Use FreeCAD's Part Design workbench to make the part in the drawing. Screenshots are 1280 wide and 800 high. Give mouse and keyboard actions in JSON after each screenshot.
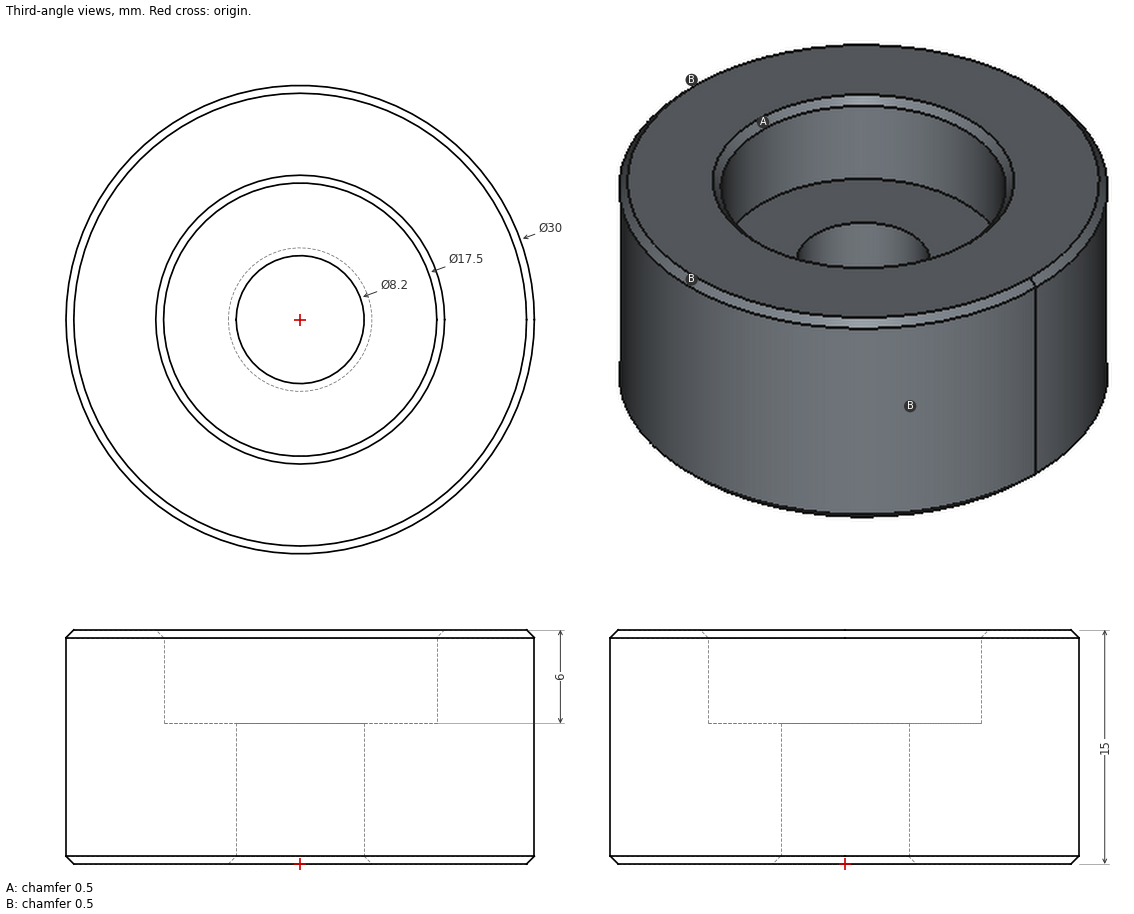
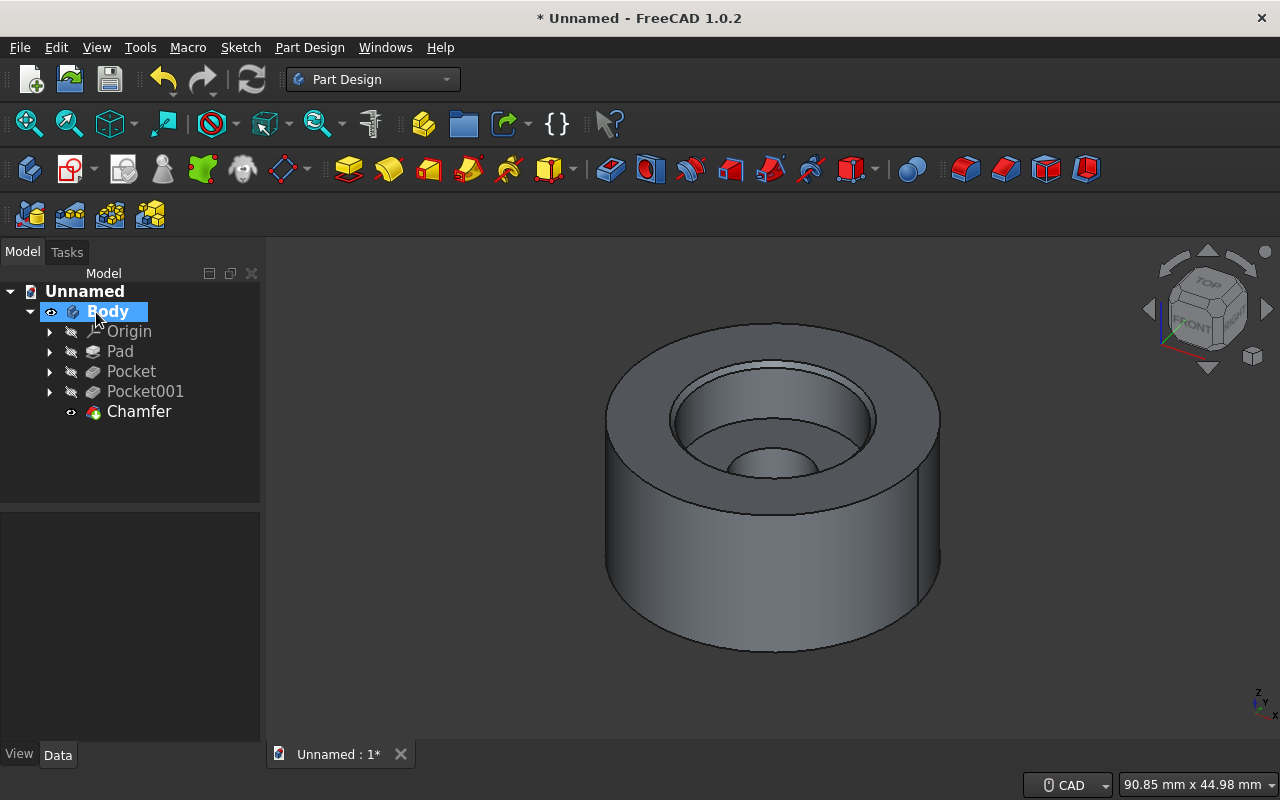
{"action": "left_click", "coordinate": [606, 428]}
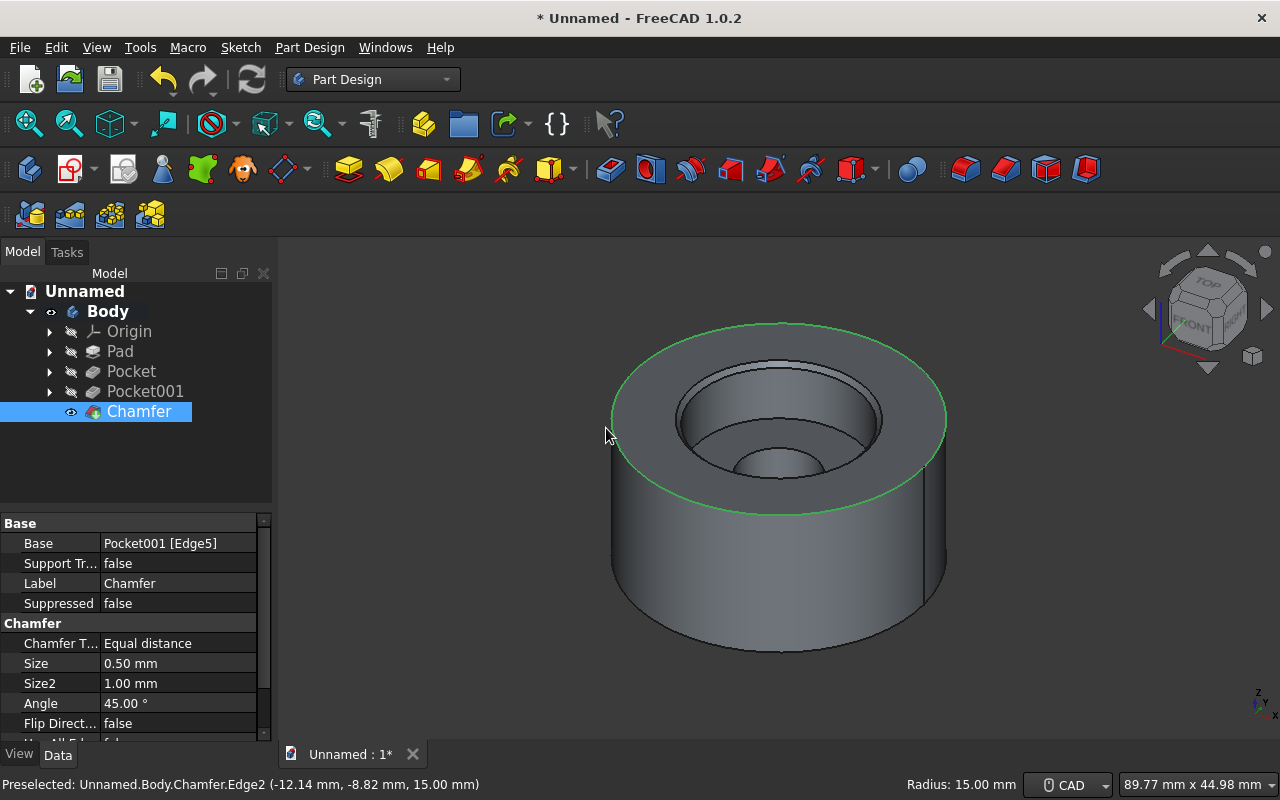
{"action": "key", "text": "0"}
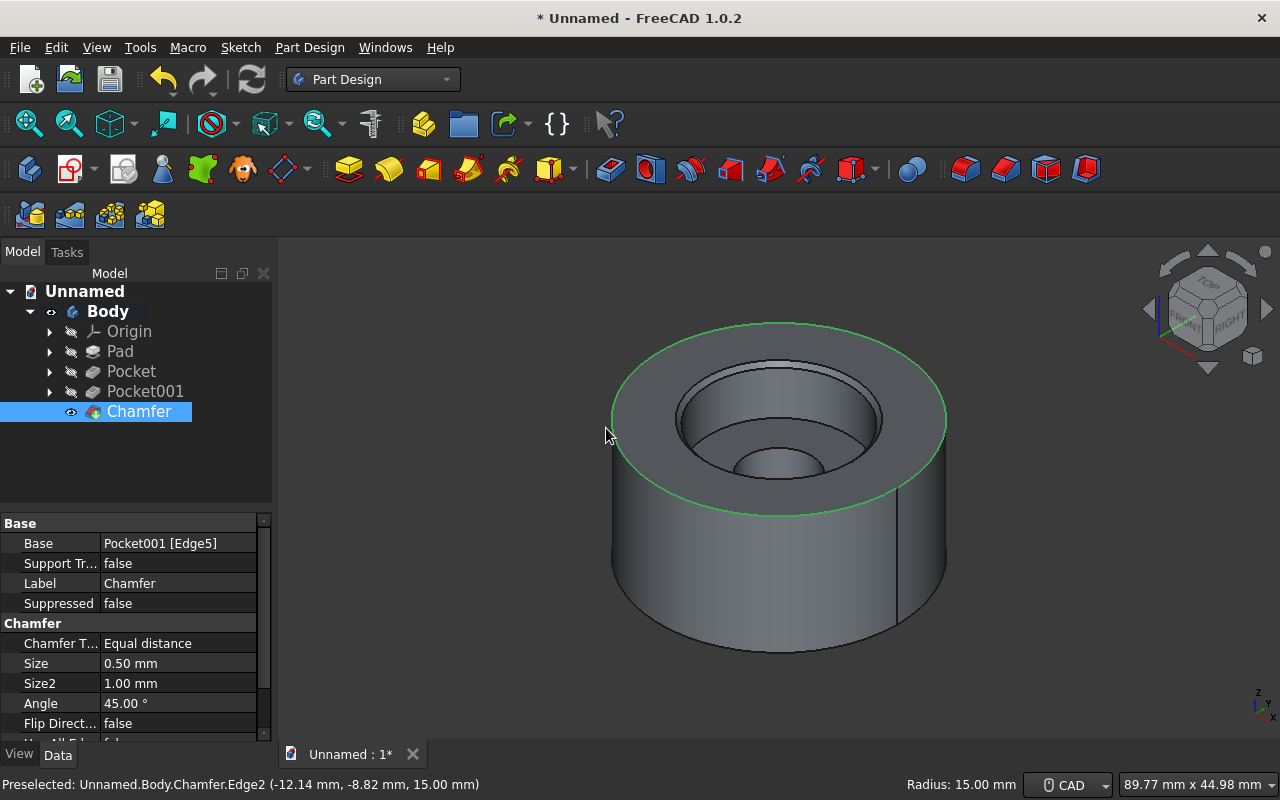
{"action": "key", "text": "2"}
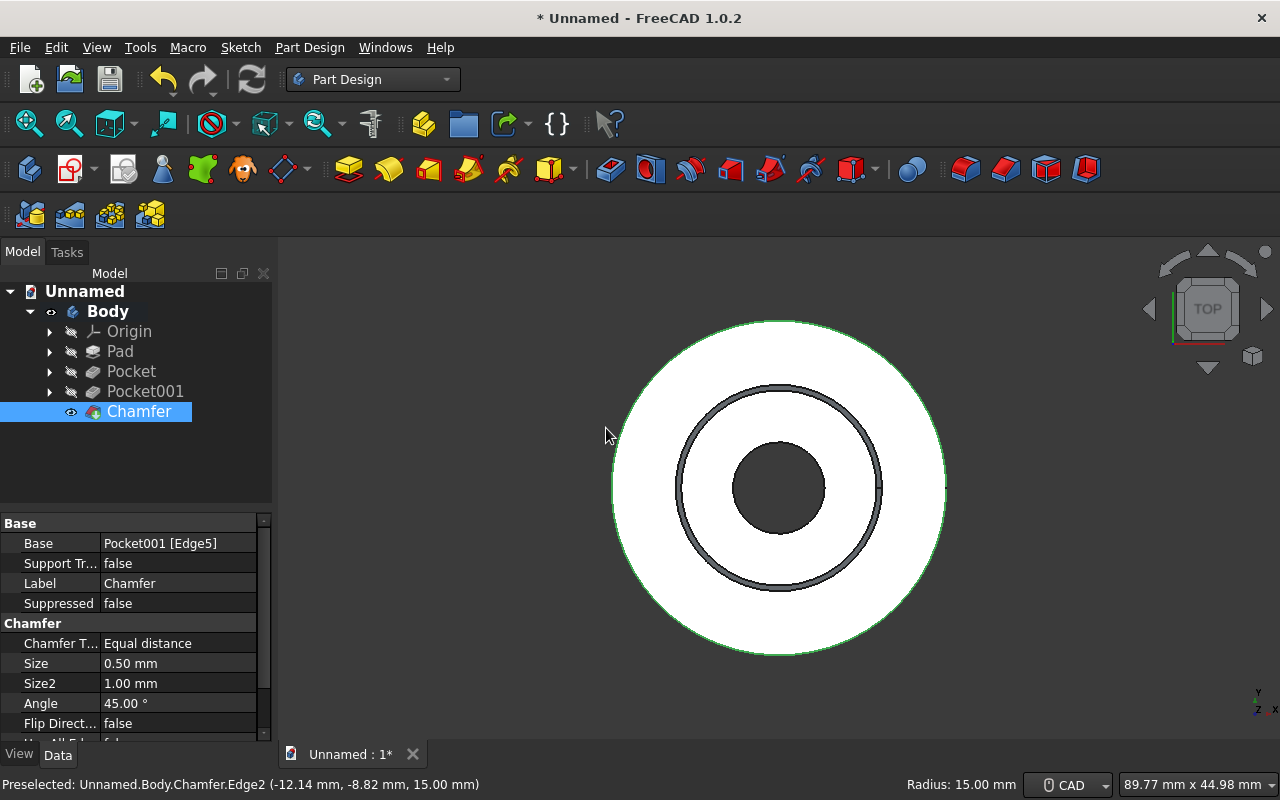
{"action": "key", "text": "1"}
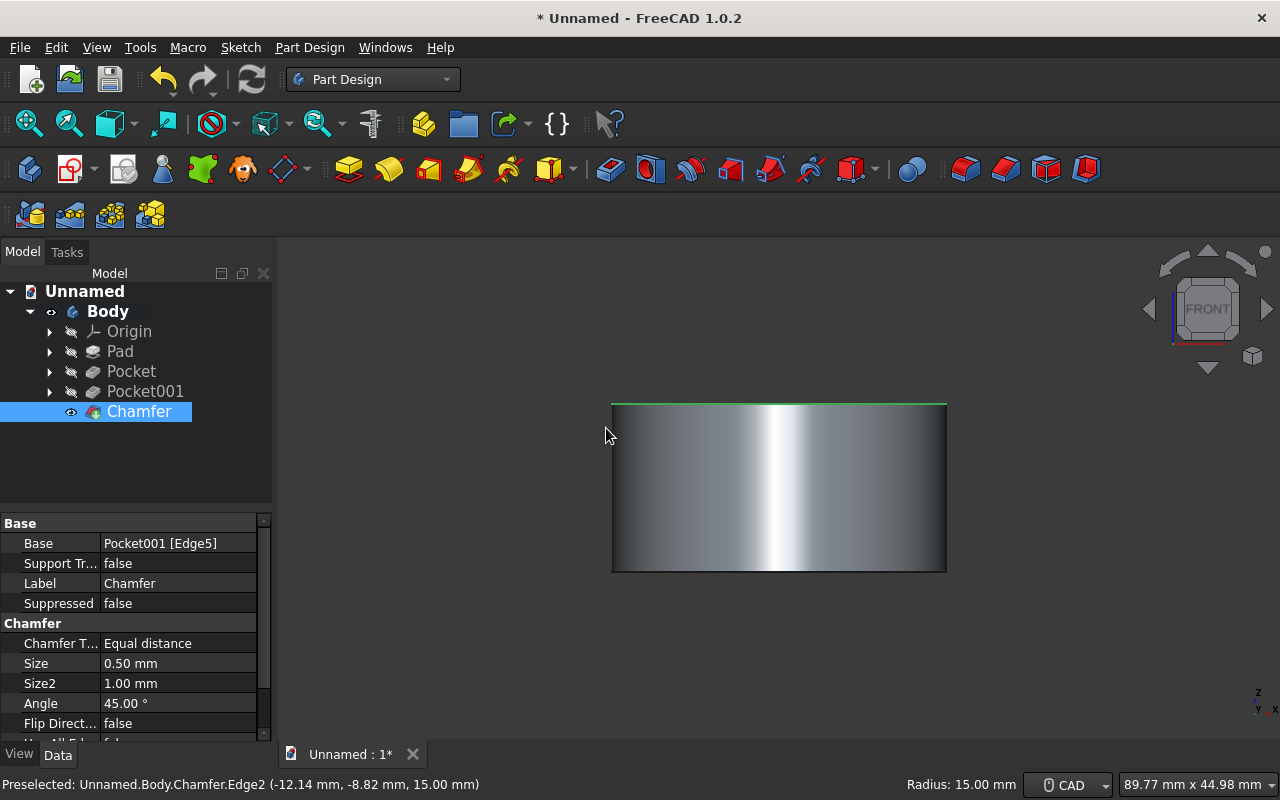
{"action": "left_click", "coordinate": [30, 124]}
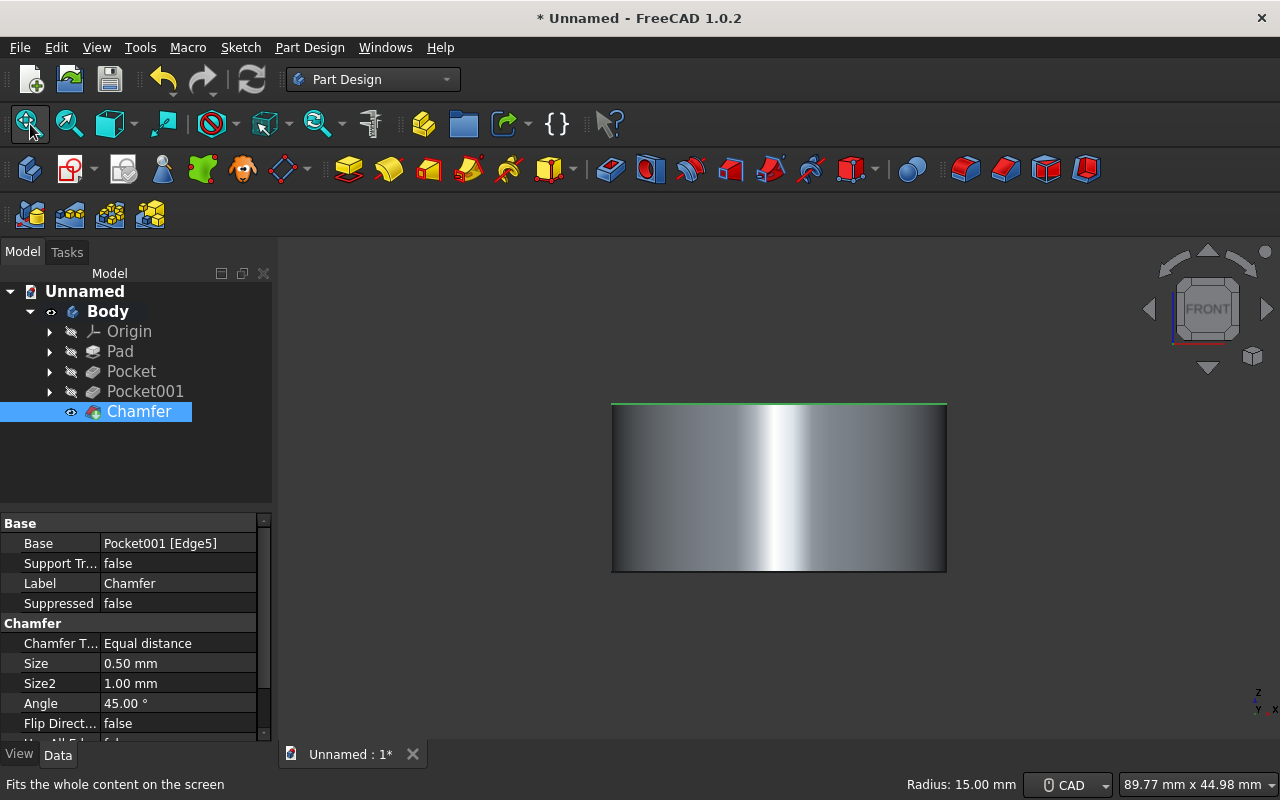
{"action": "left_click", "coordinate": [643, 571], "text": "ctrl"}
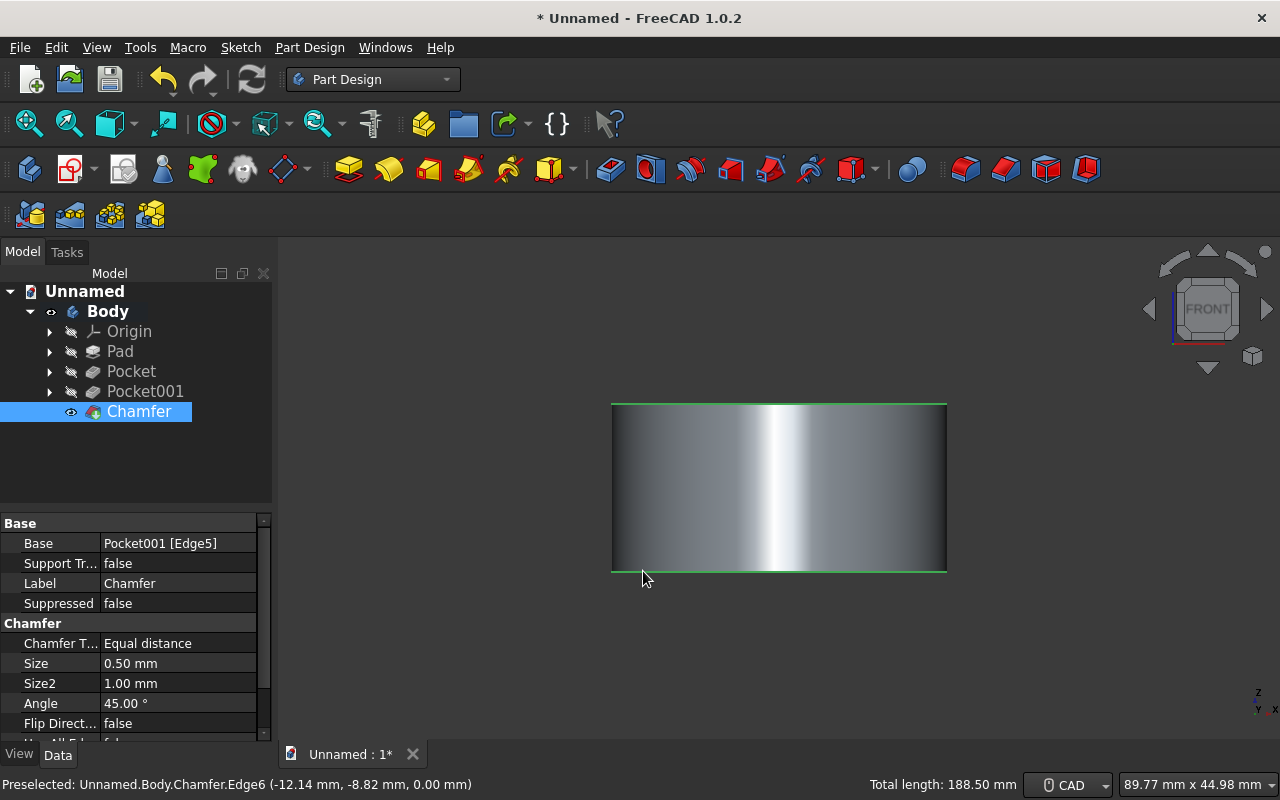
{"action": "key", "text": "3"}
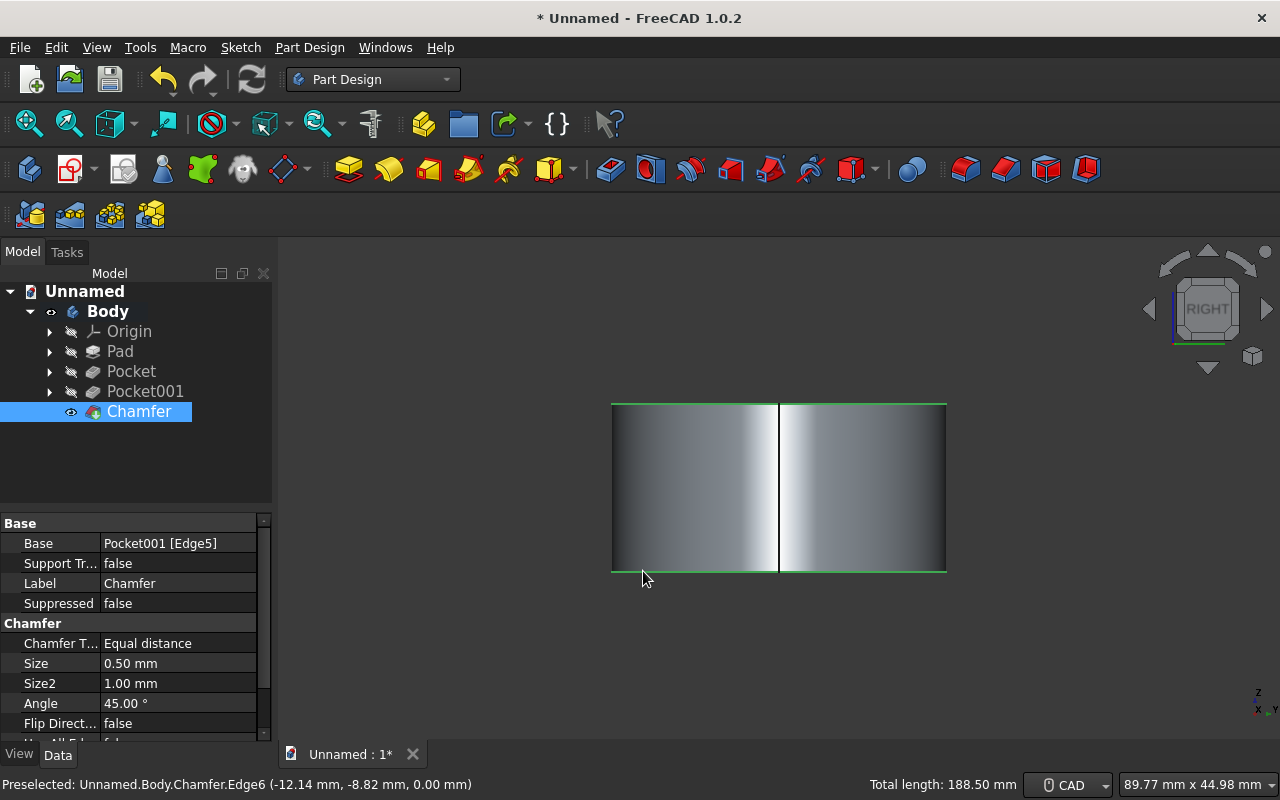
{"action": "left_click", "coordinate": [30, 124]}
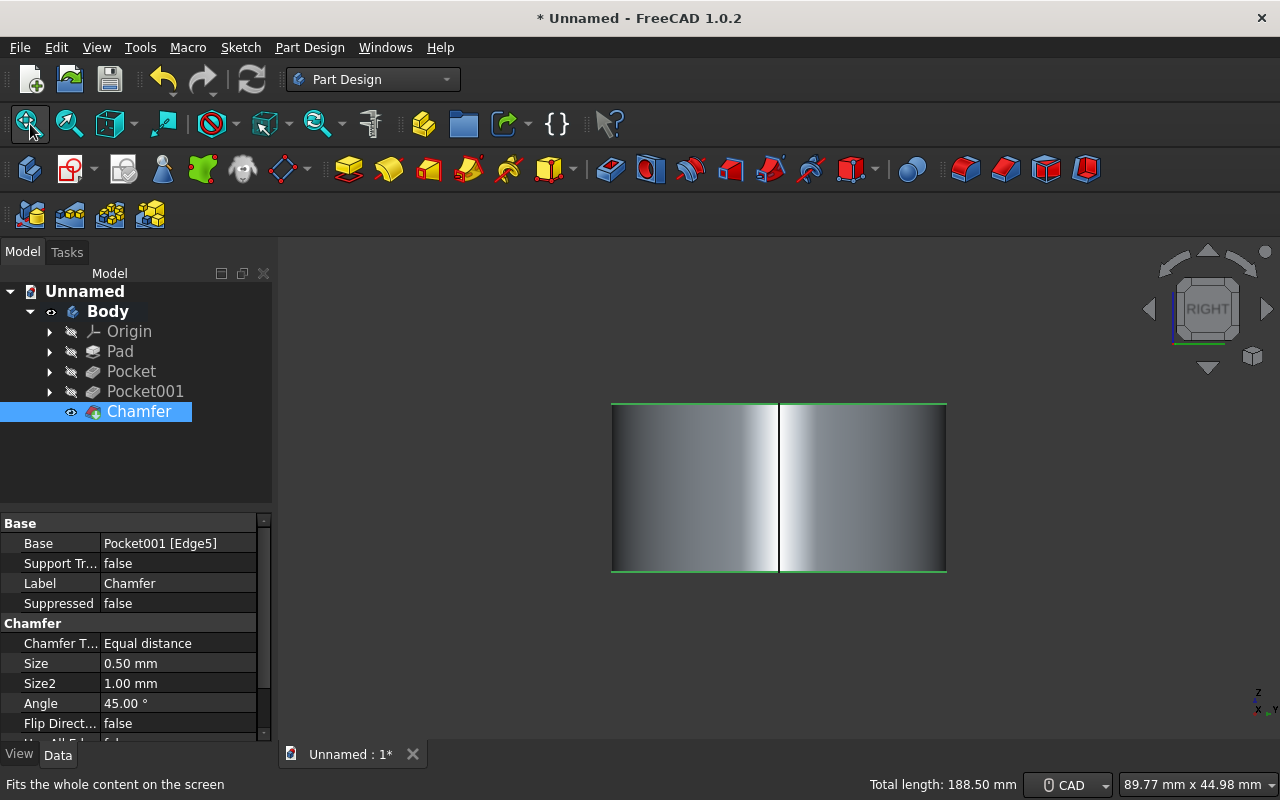
{"action": "key", "text": "5"}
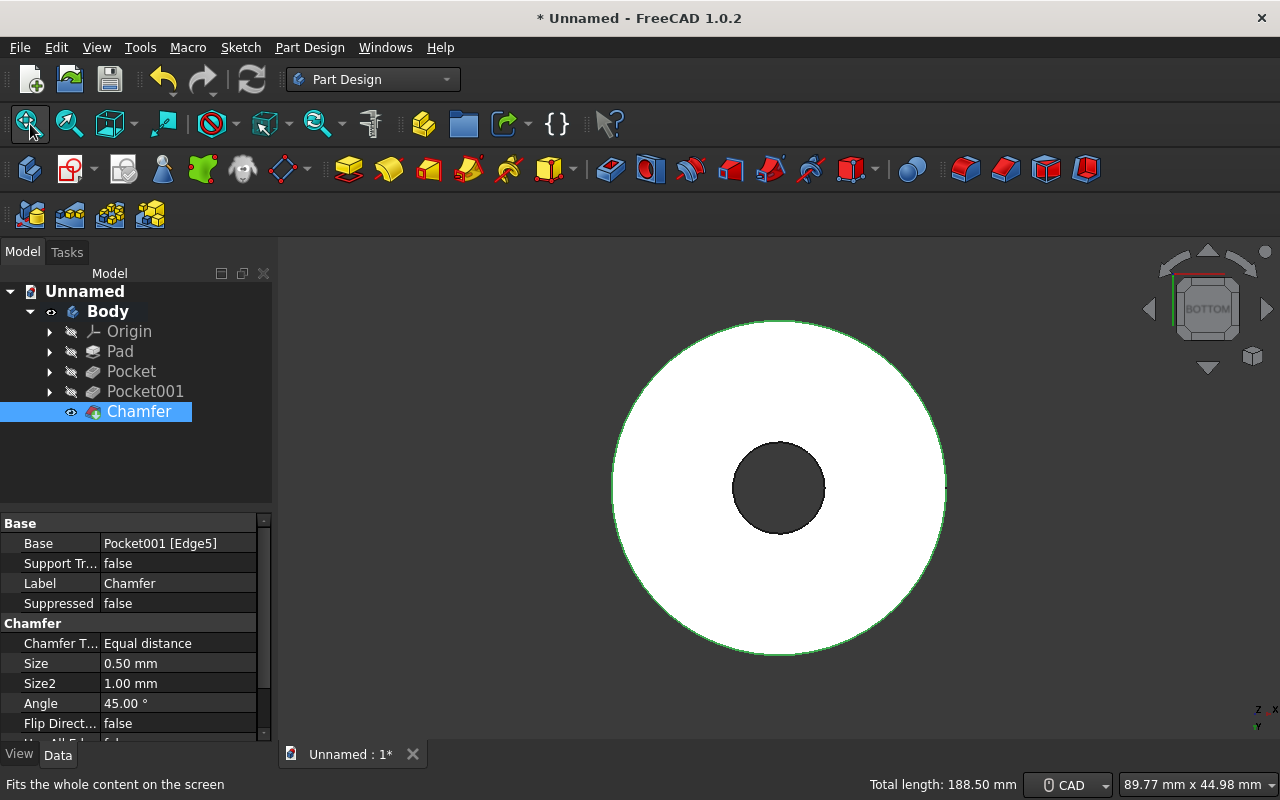
{"action": "left_click", "coordinate": [742, 514], "text": "ctrl"}